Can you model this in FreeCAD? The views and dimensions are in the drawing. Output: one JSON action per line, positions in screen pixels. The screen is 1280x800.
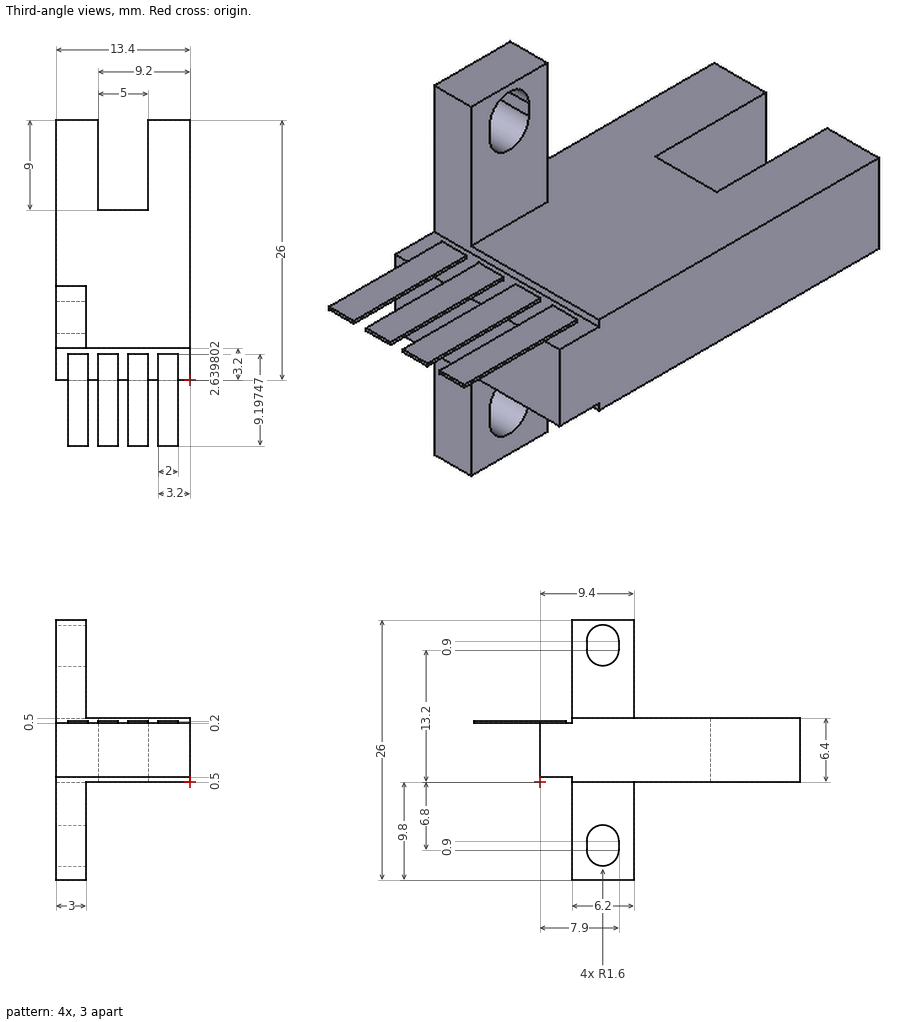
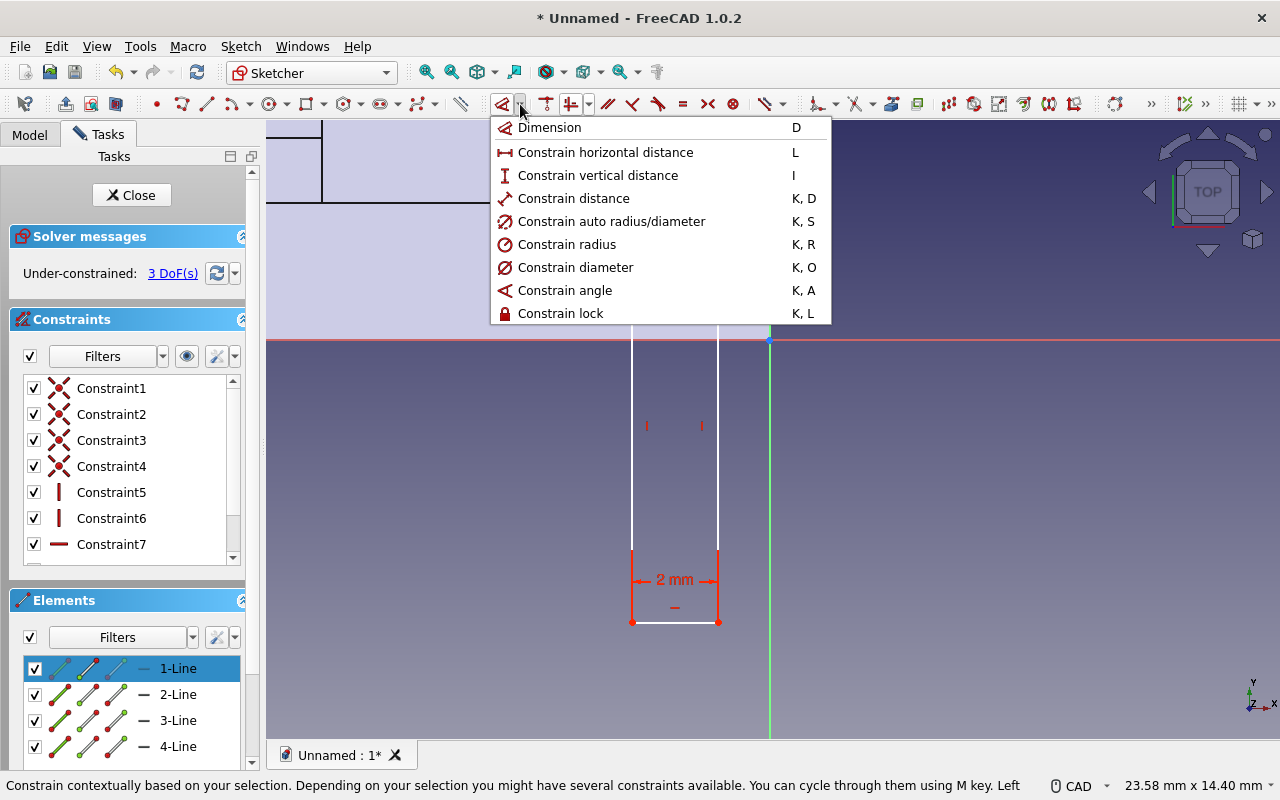
{"action": "left_click", "coordinate": [661, 152]}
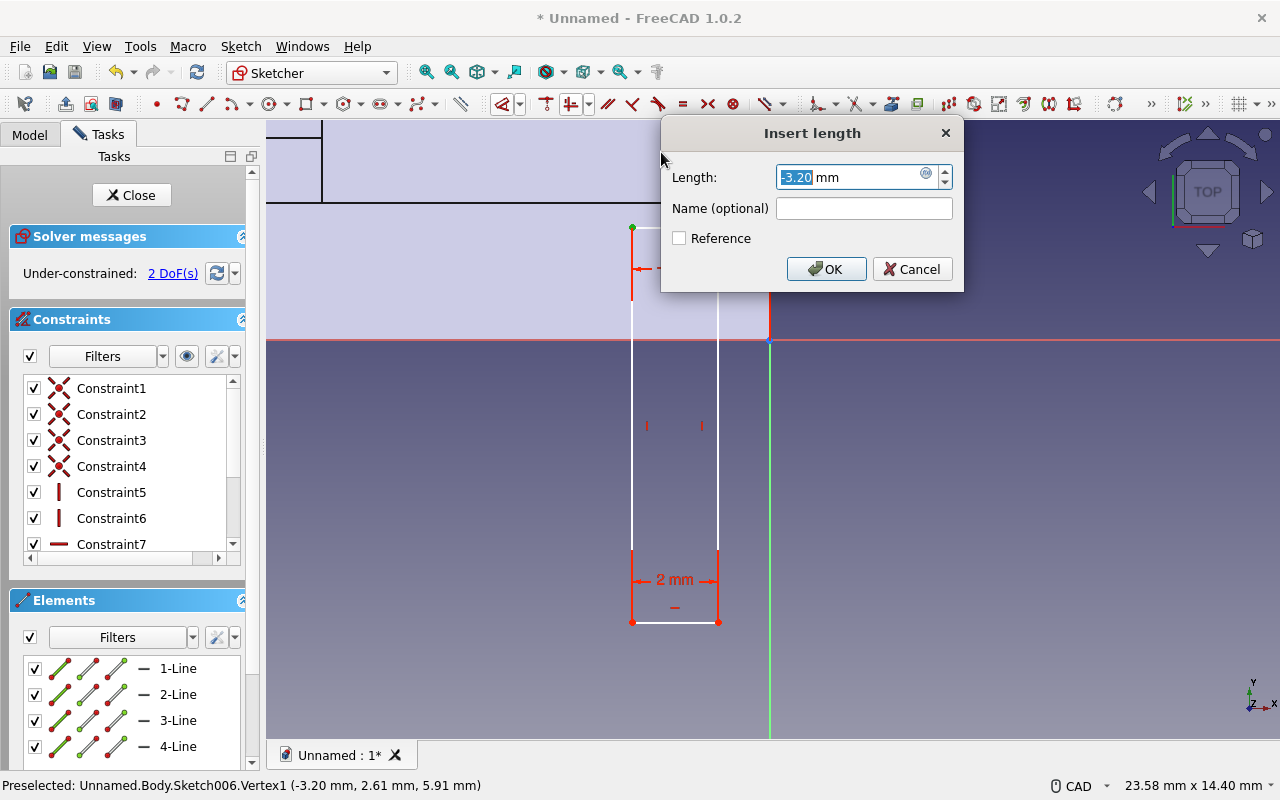
{"action": "type", "text": "-3.2"}
{"action": "key", "text": "Return"}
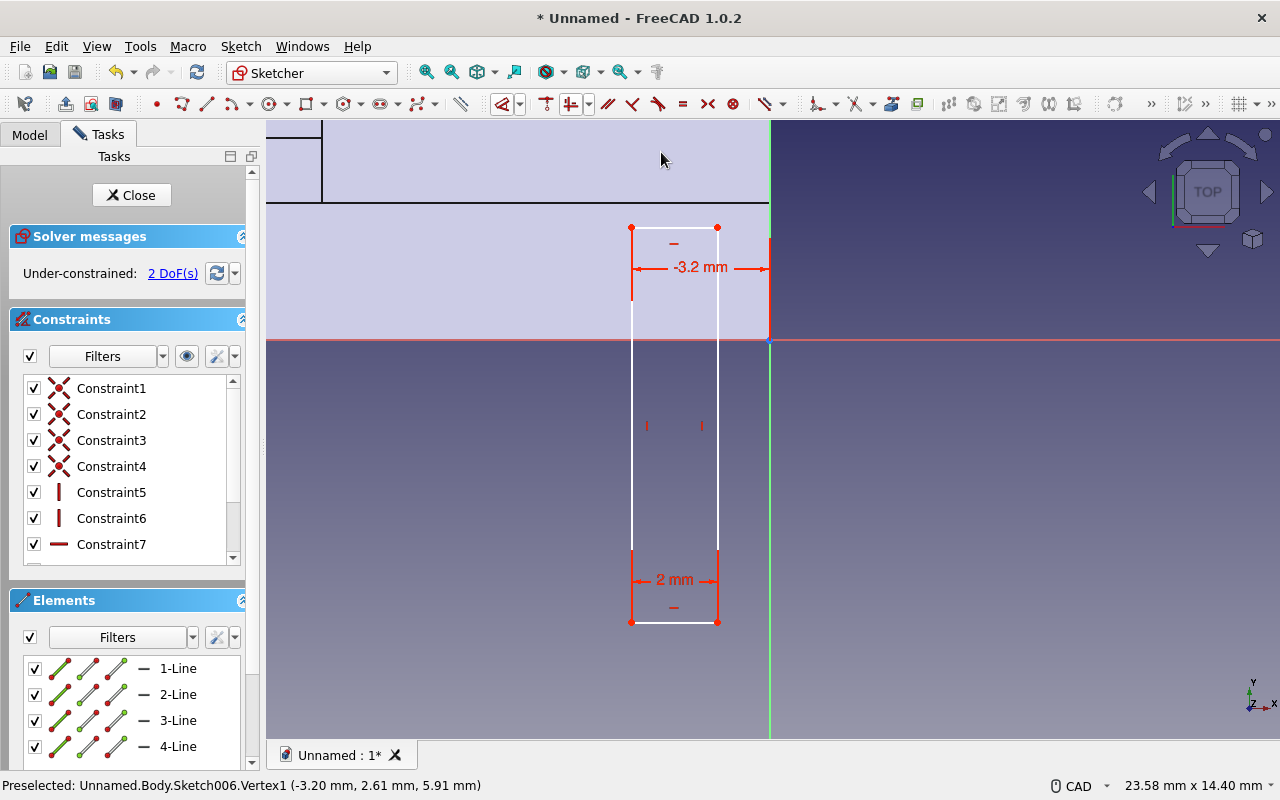
{"action": "left_click", "coordinate": [632, 504]}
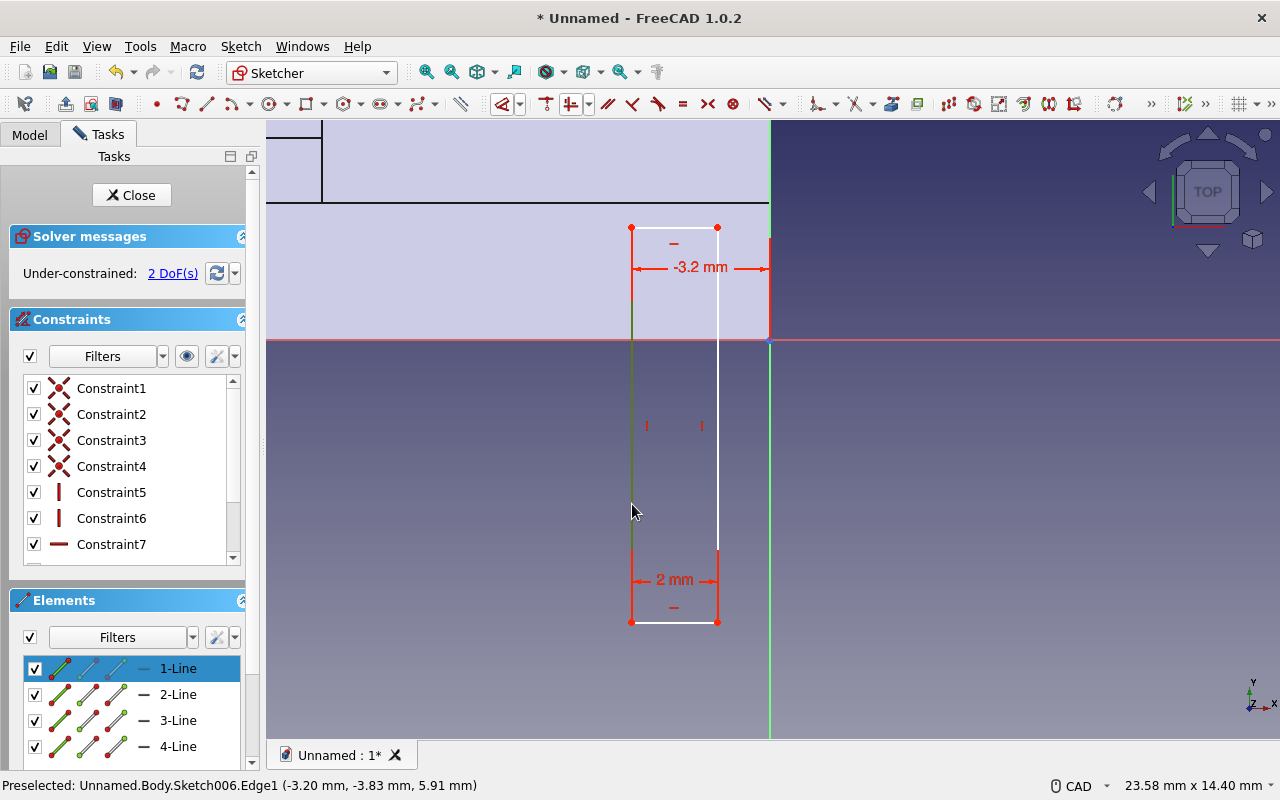
{"action": "left_click", "coordinate": [520, 104]}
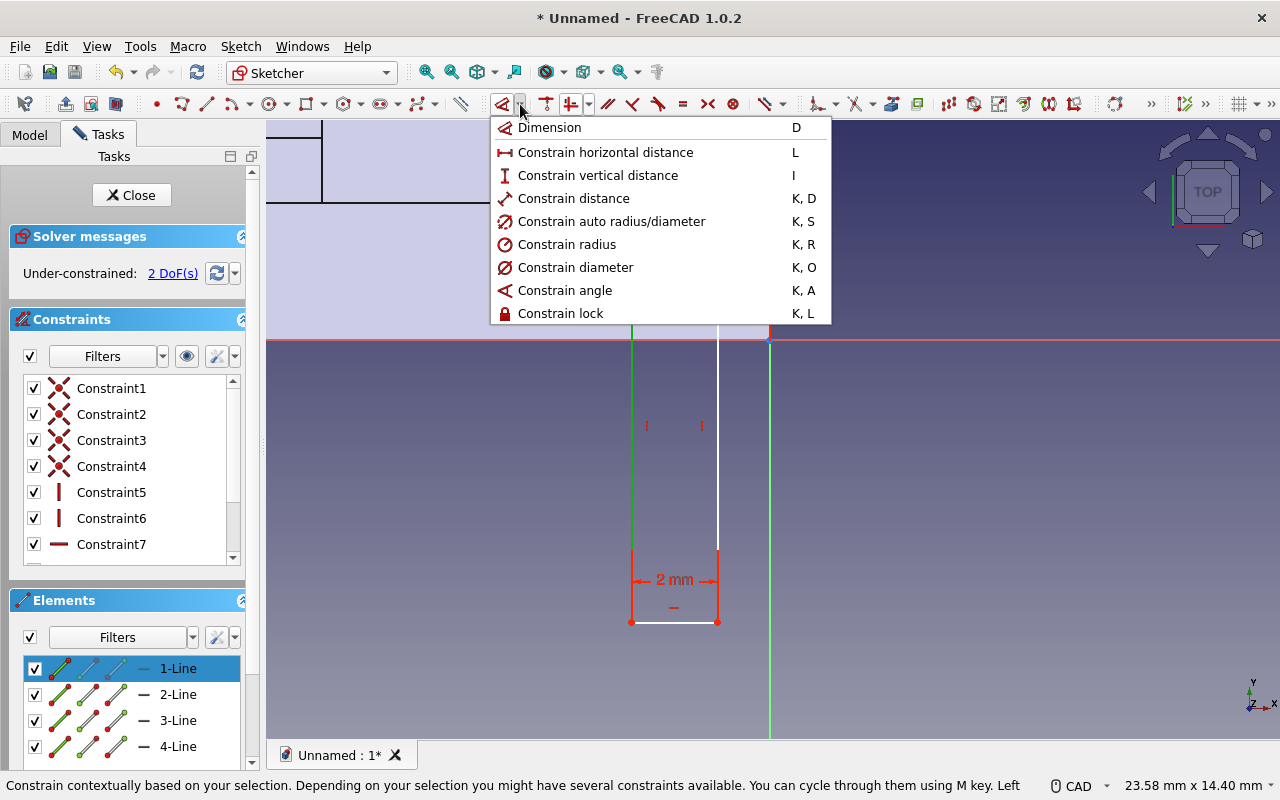
{"action": "left_click", "coordinate": [661, 176]}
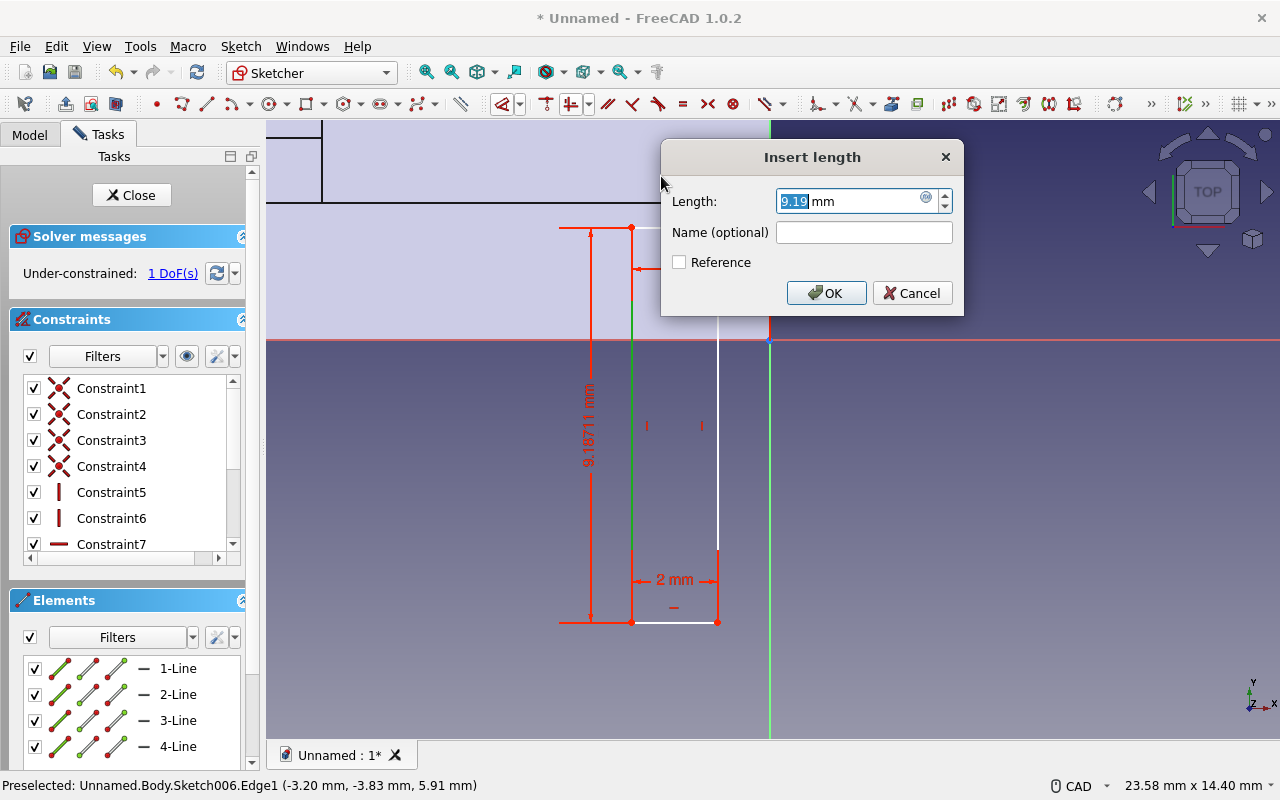
{"action": "type", "text": "9.19747"}
{"action": "key", "text": "Return"}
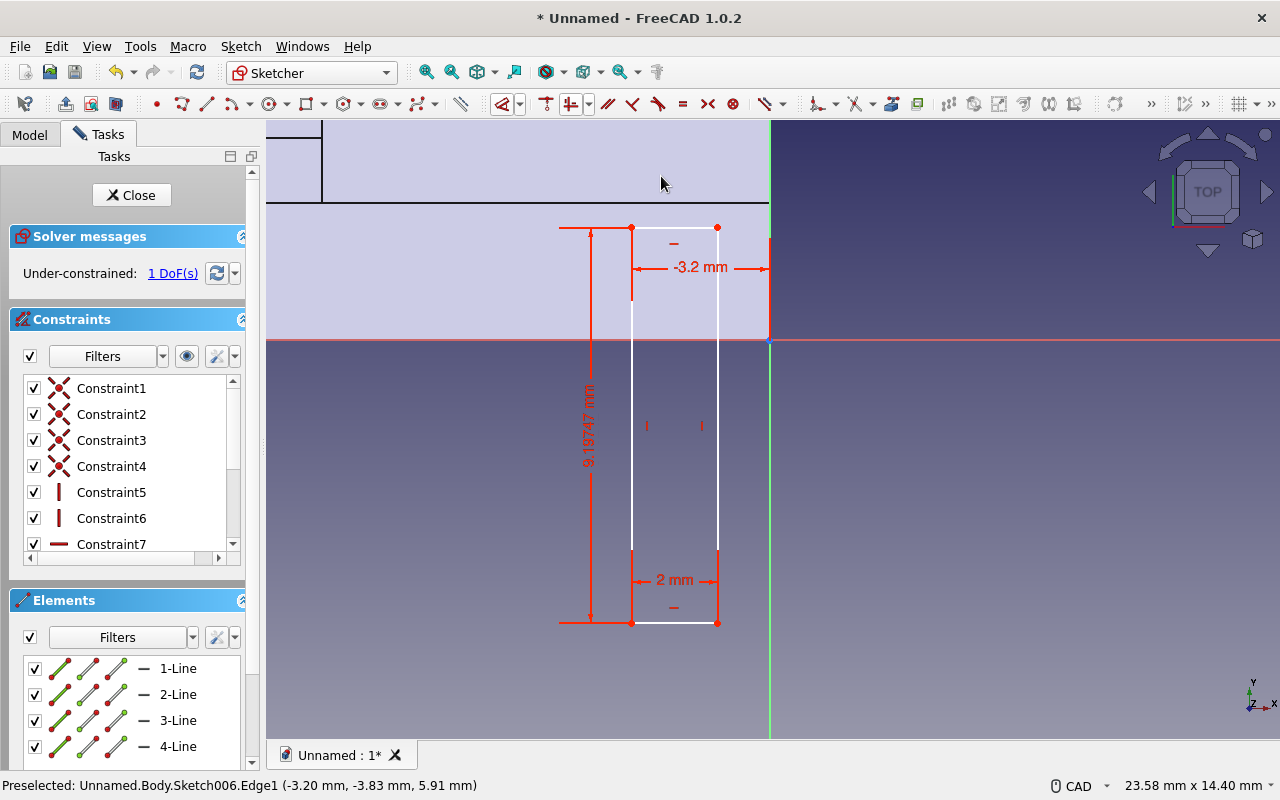
{"action": "left_click", "coordinate": [632, 228]}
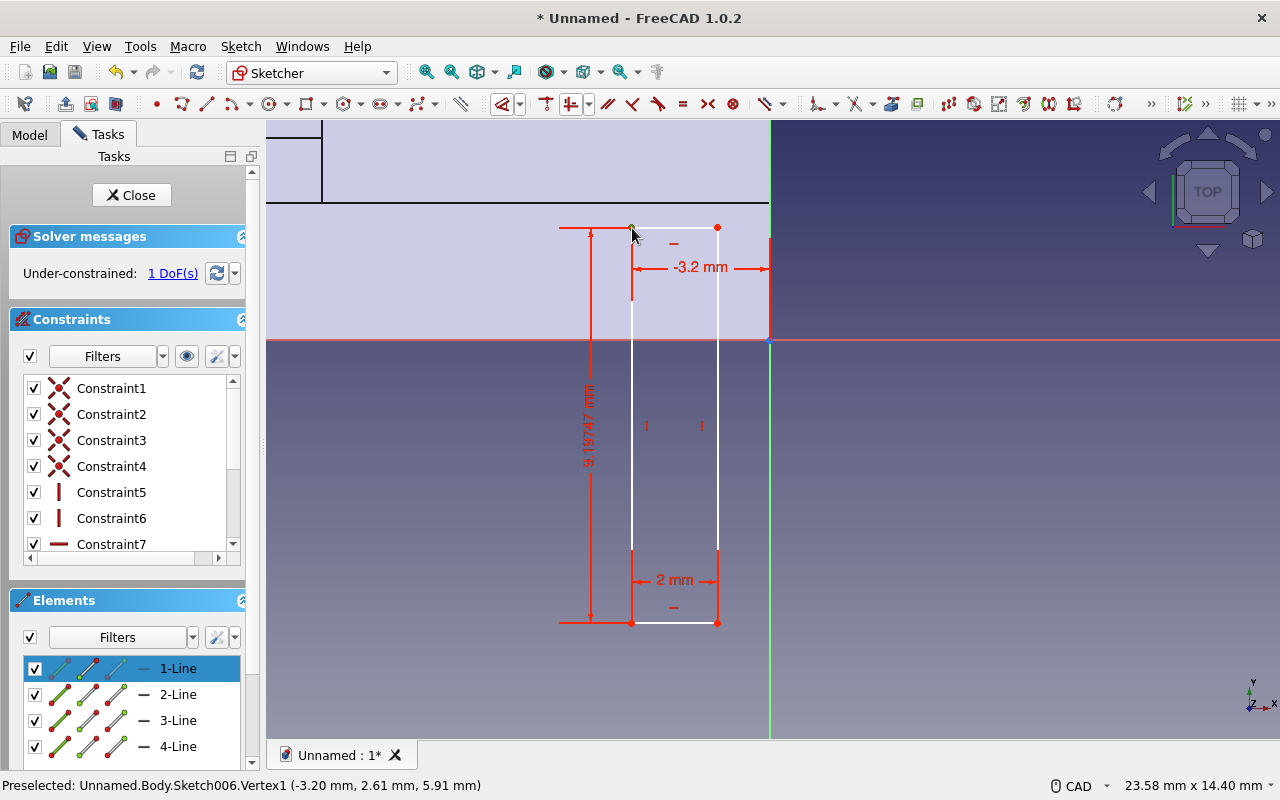
{"action": "key", "text": "i"}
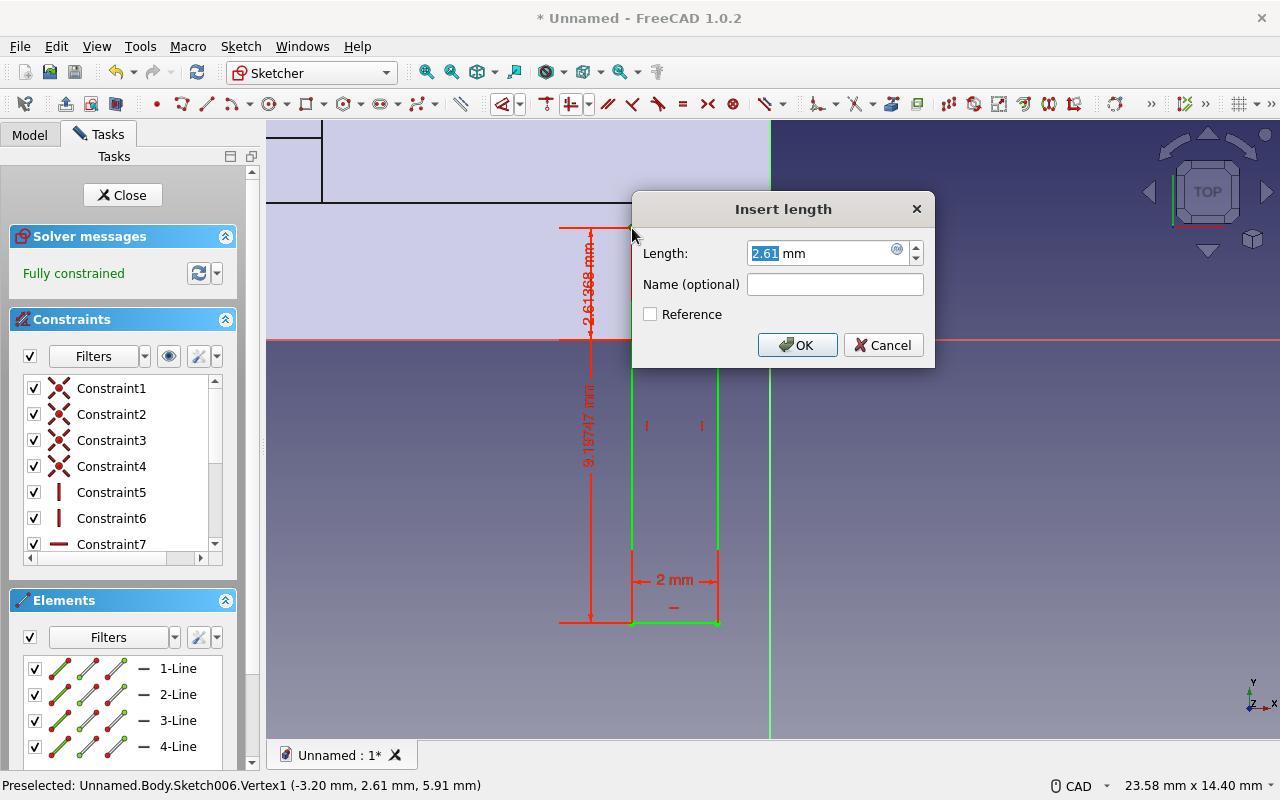
{"action": "type", "text": "2.639802"}
{"action": "key", "text": "Return"}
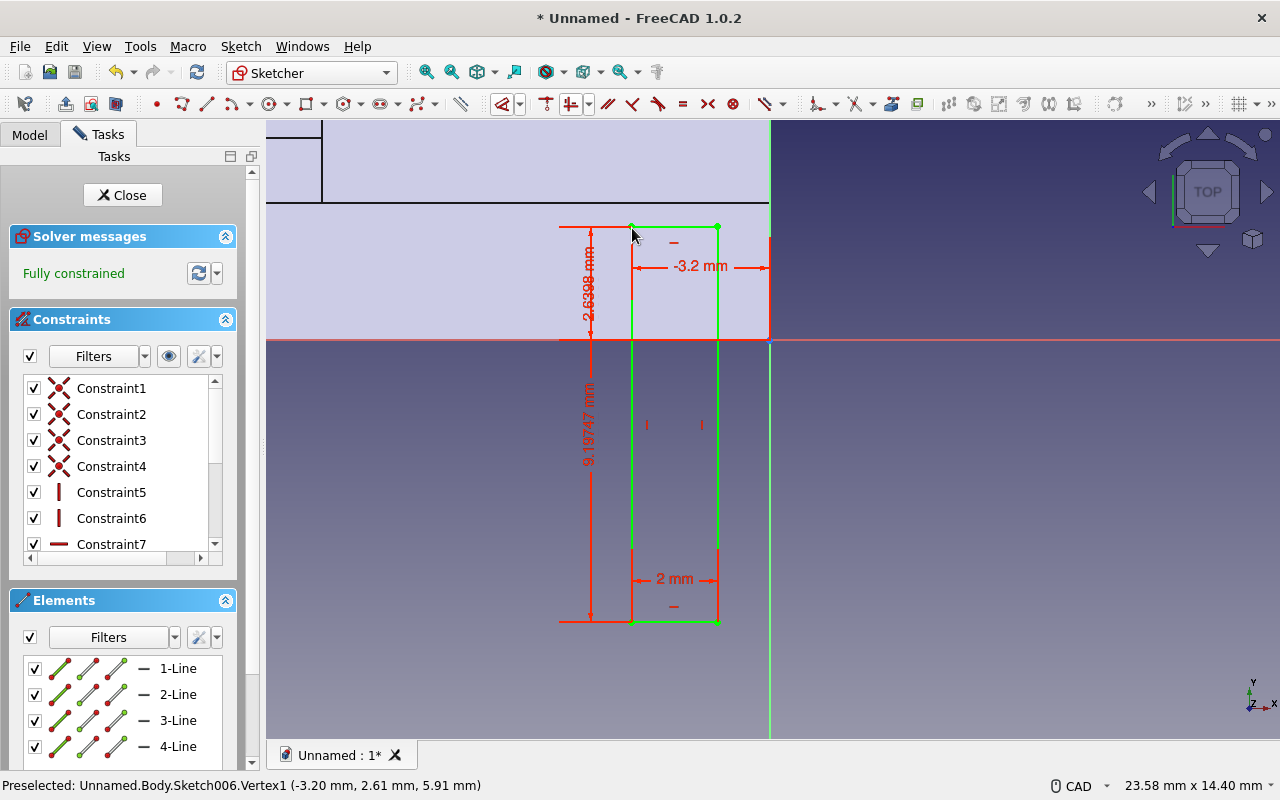
{"action": "left_click", "coordinate": [123, 195]}